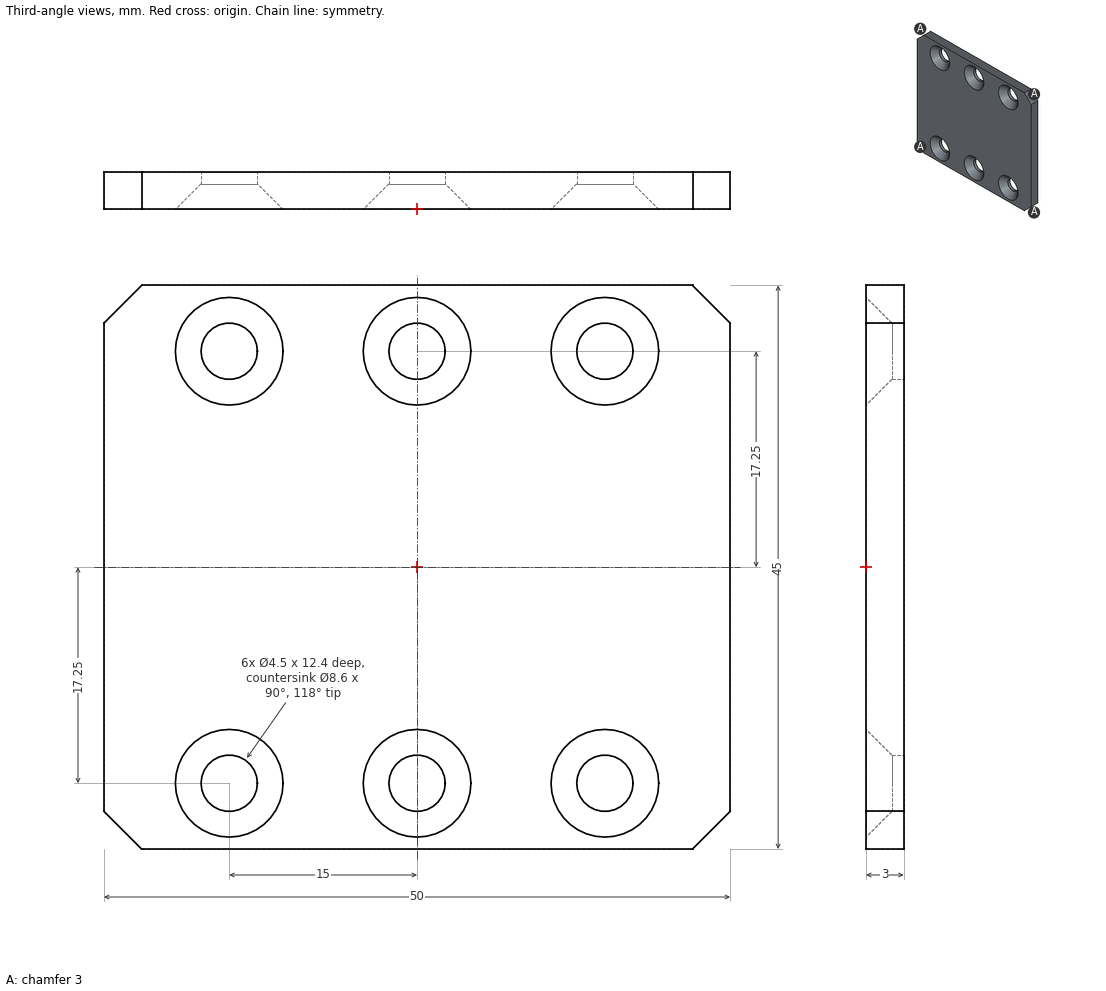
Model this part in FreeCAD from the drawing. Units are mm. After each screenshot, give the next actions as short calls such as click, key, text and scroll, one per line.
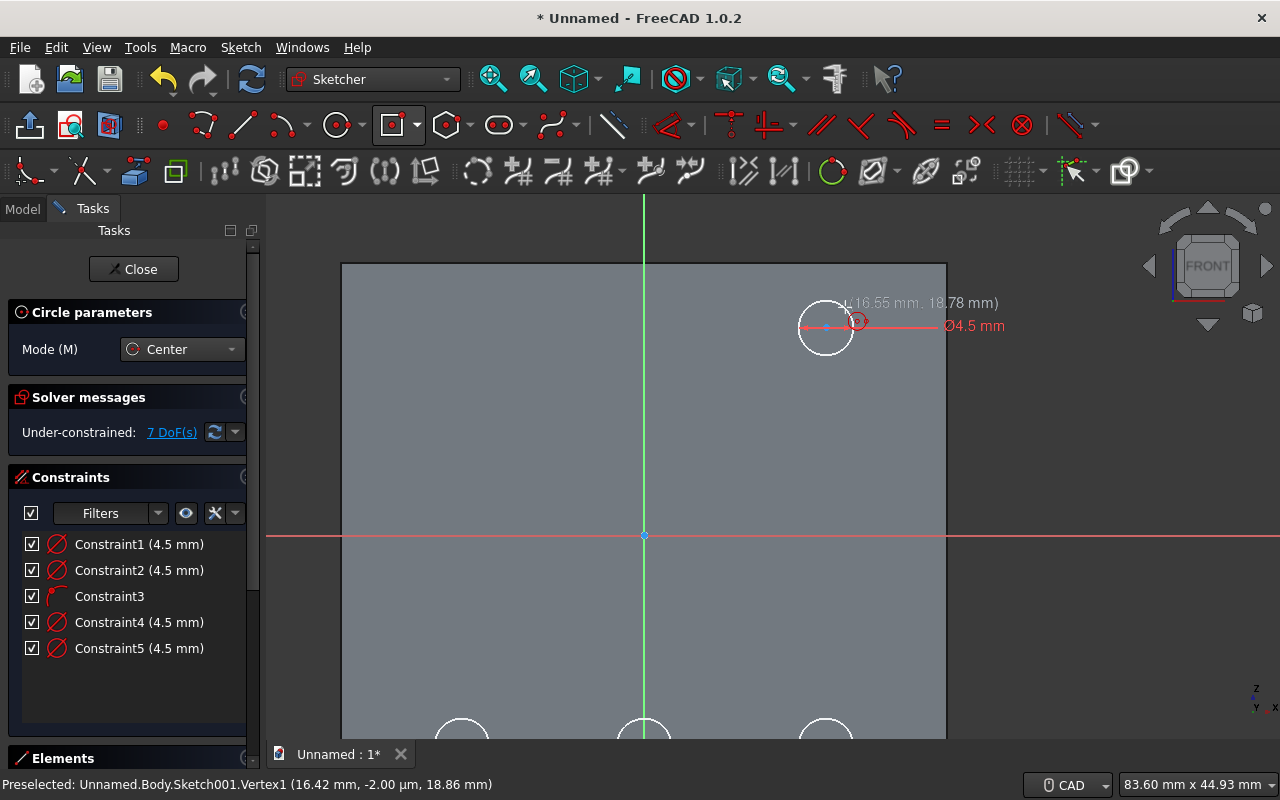
click(644, 327)
move(664, 307)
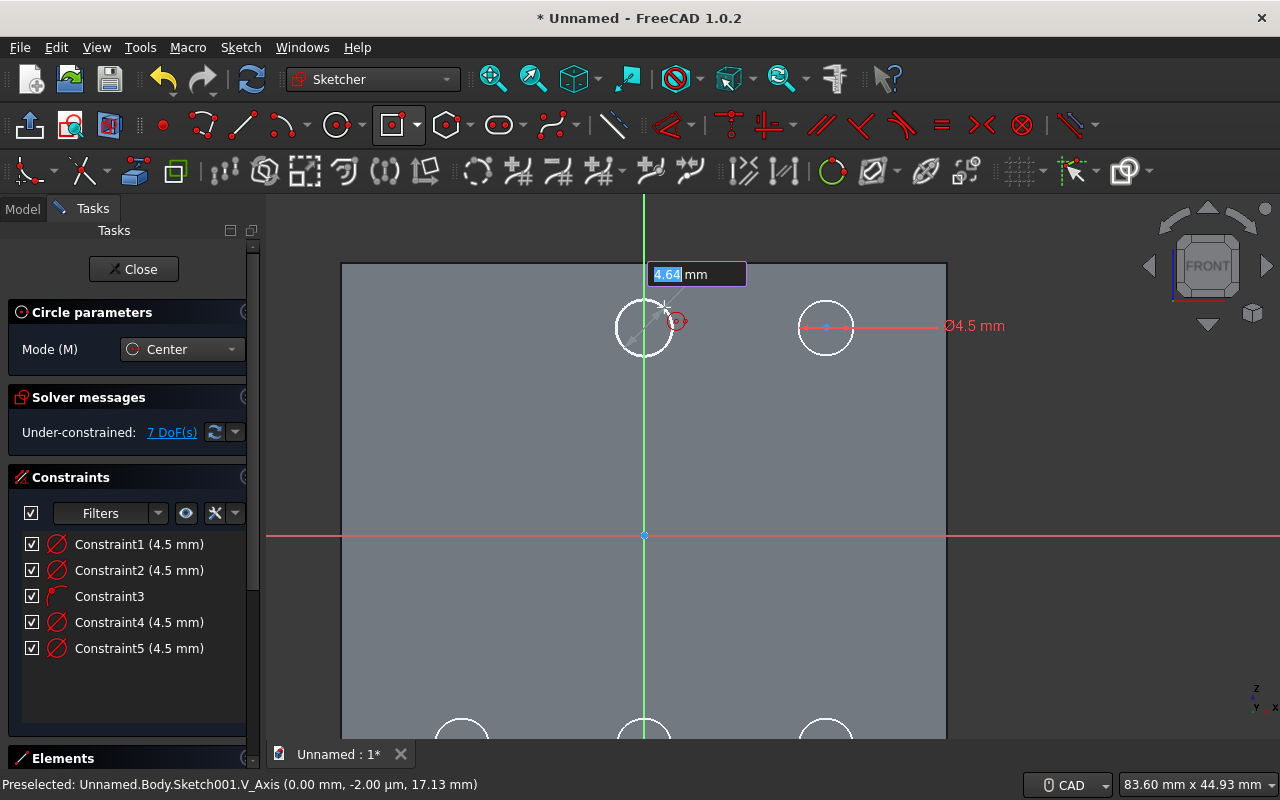
text(4.5)
key(Return)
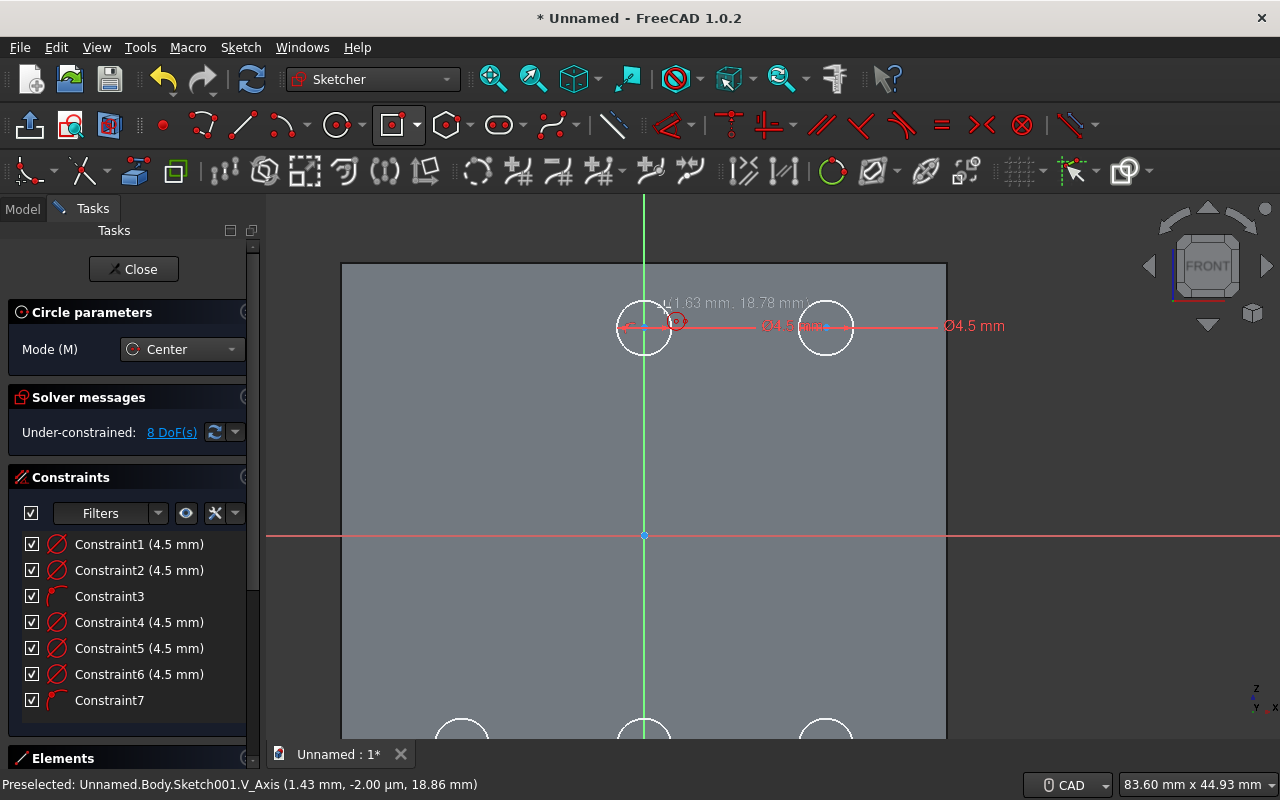
click(462, 327)
move(482, 307)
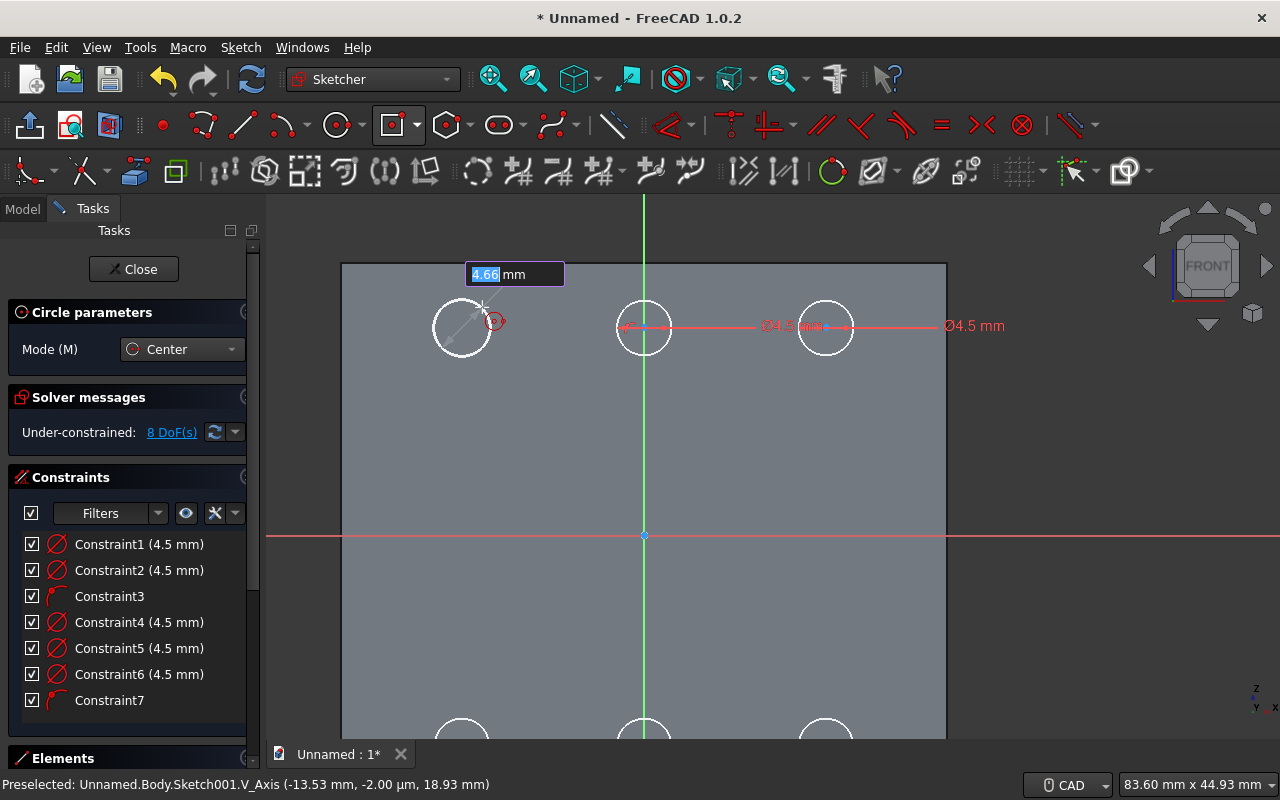
text(4.5)
key(Return)
key(Escape)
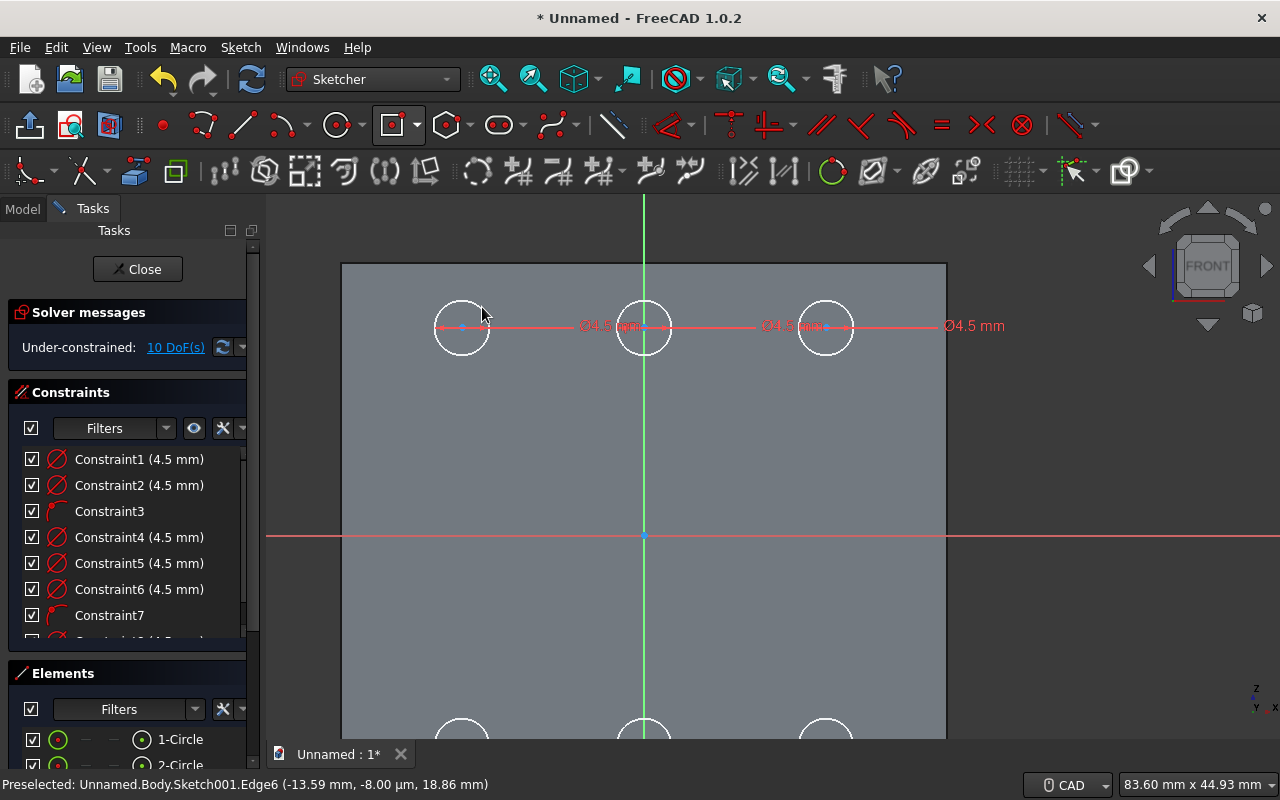
scroll(827, 326, down, 2)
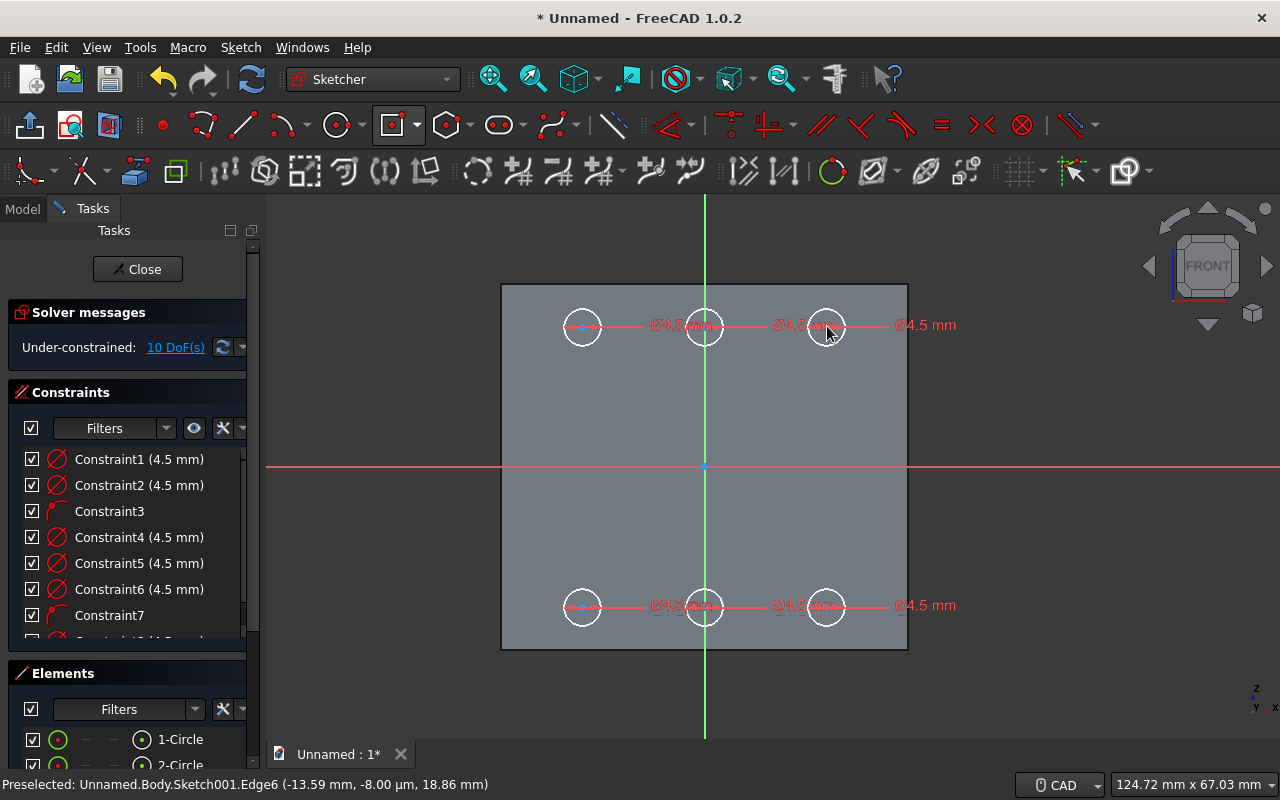
click(582, 608)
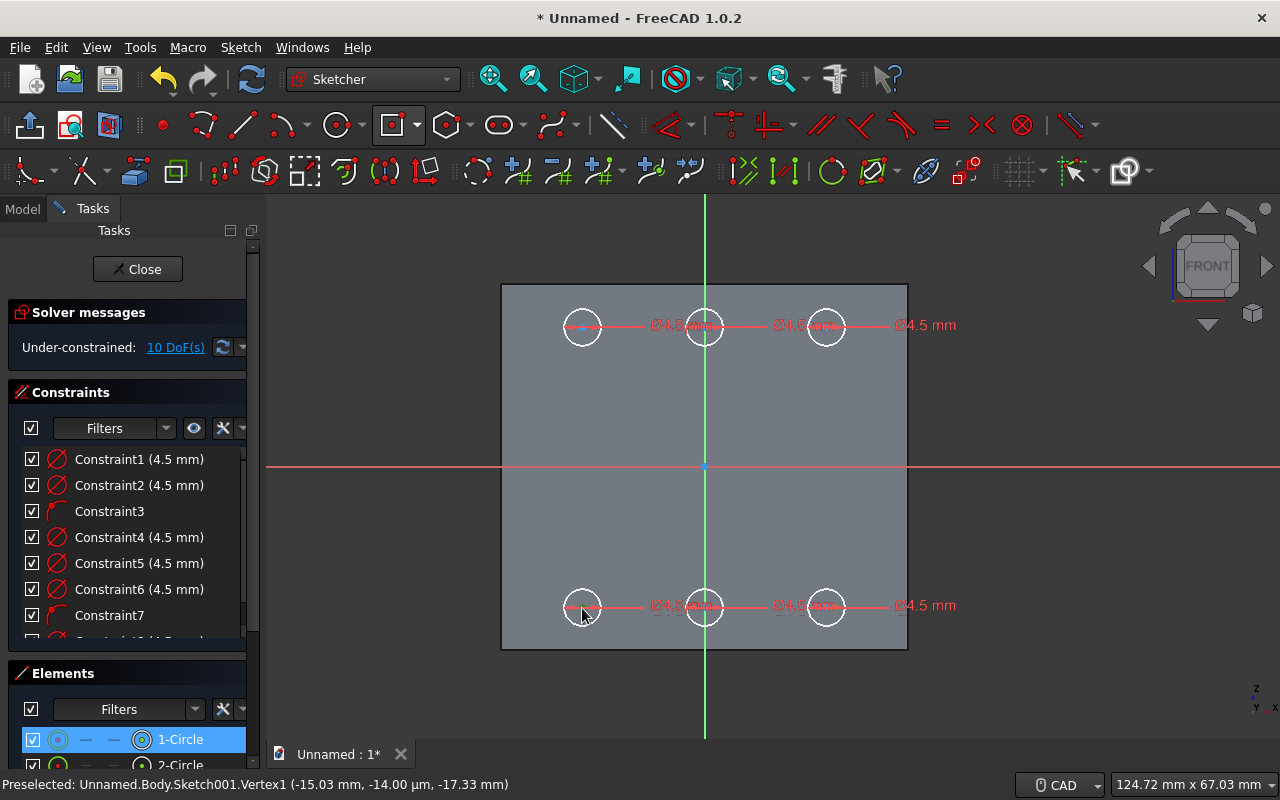
click(826, 608)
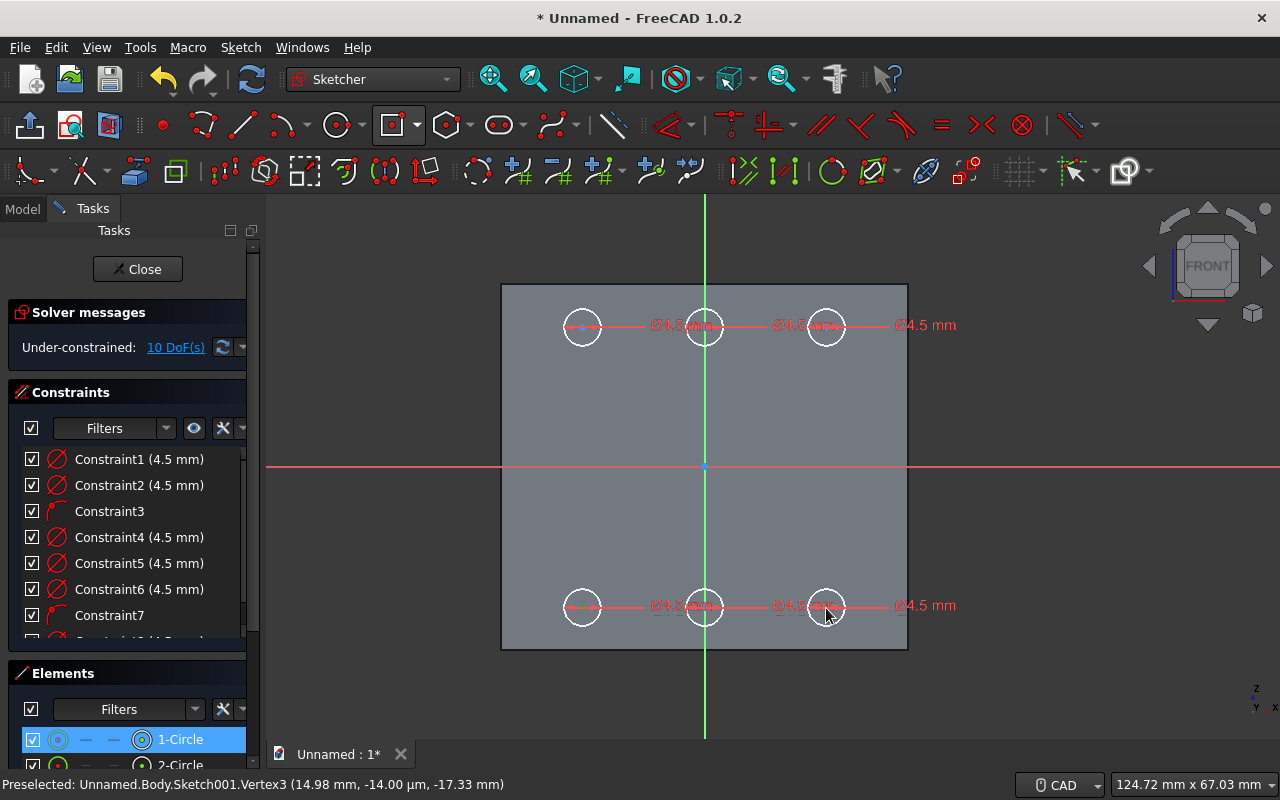
click(705, 676)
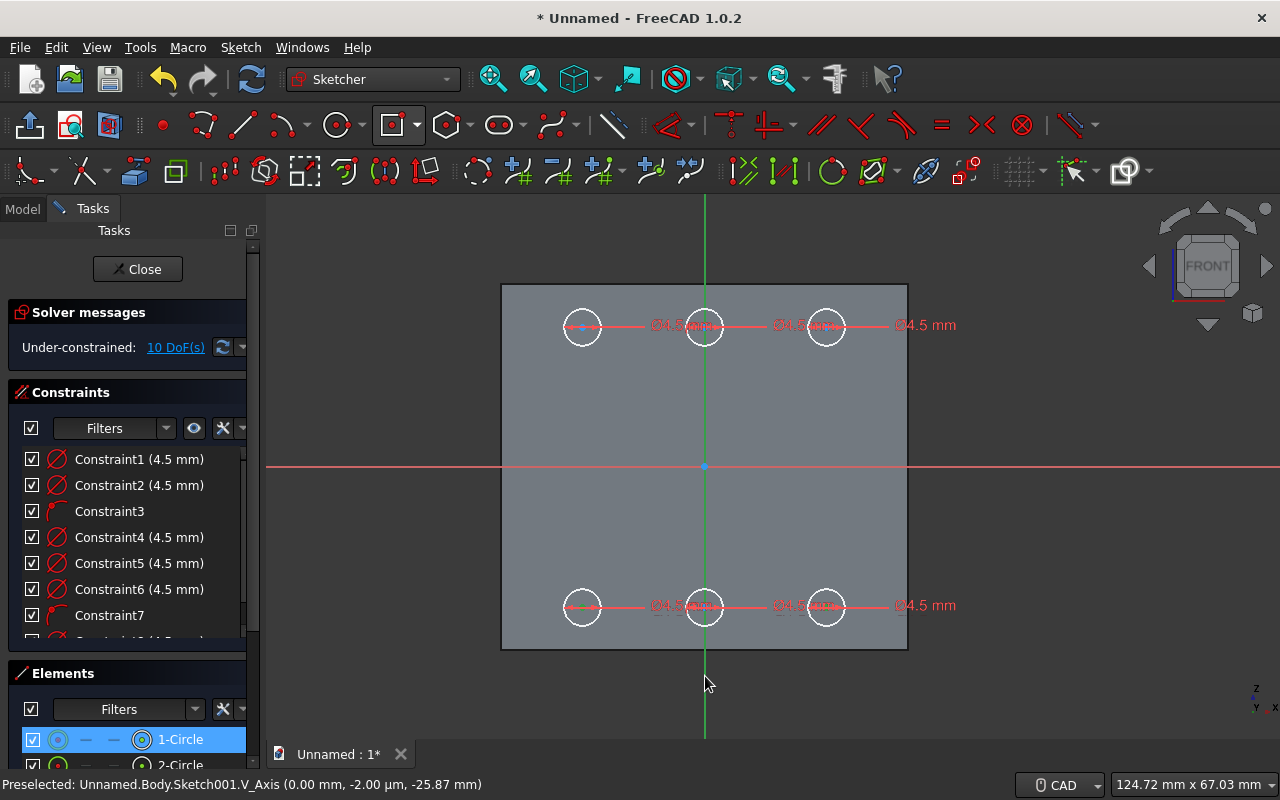
click(982, 126)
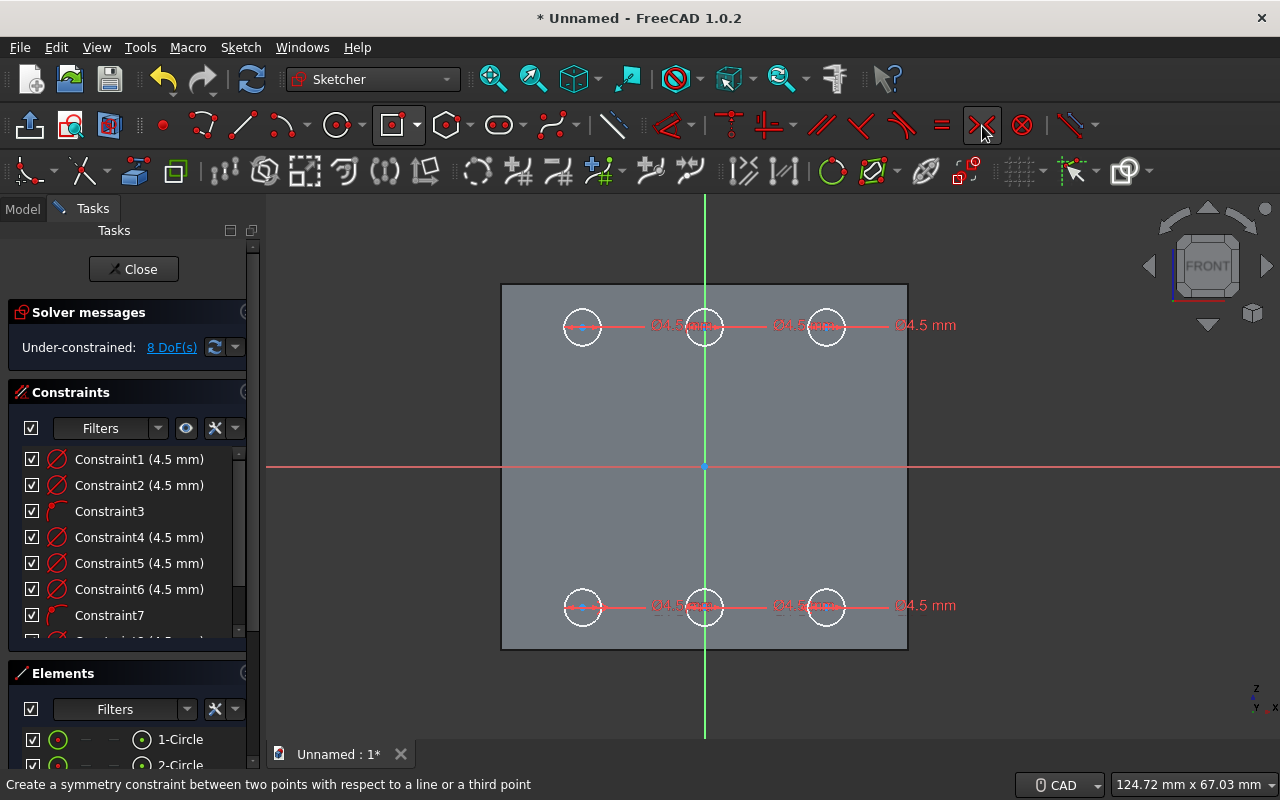
click(826, 608)